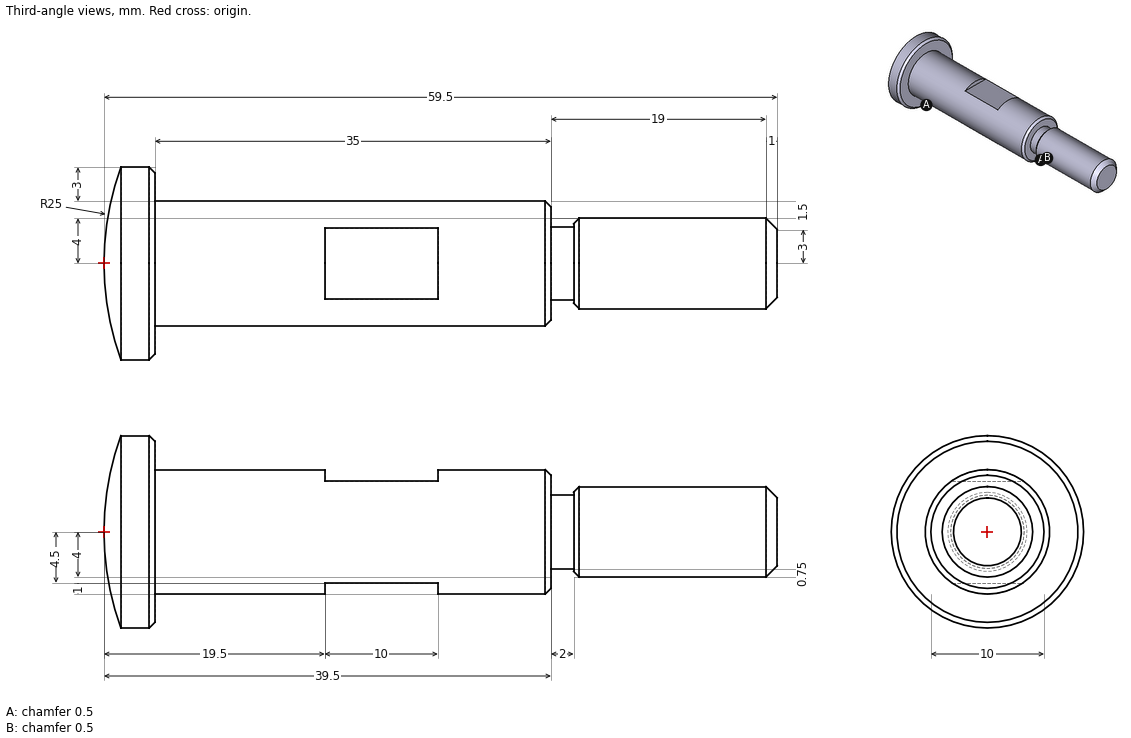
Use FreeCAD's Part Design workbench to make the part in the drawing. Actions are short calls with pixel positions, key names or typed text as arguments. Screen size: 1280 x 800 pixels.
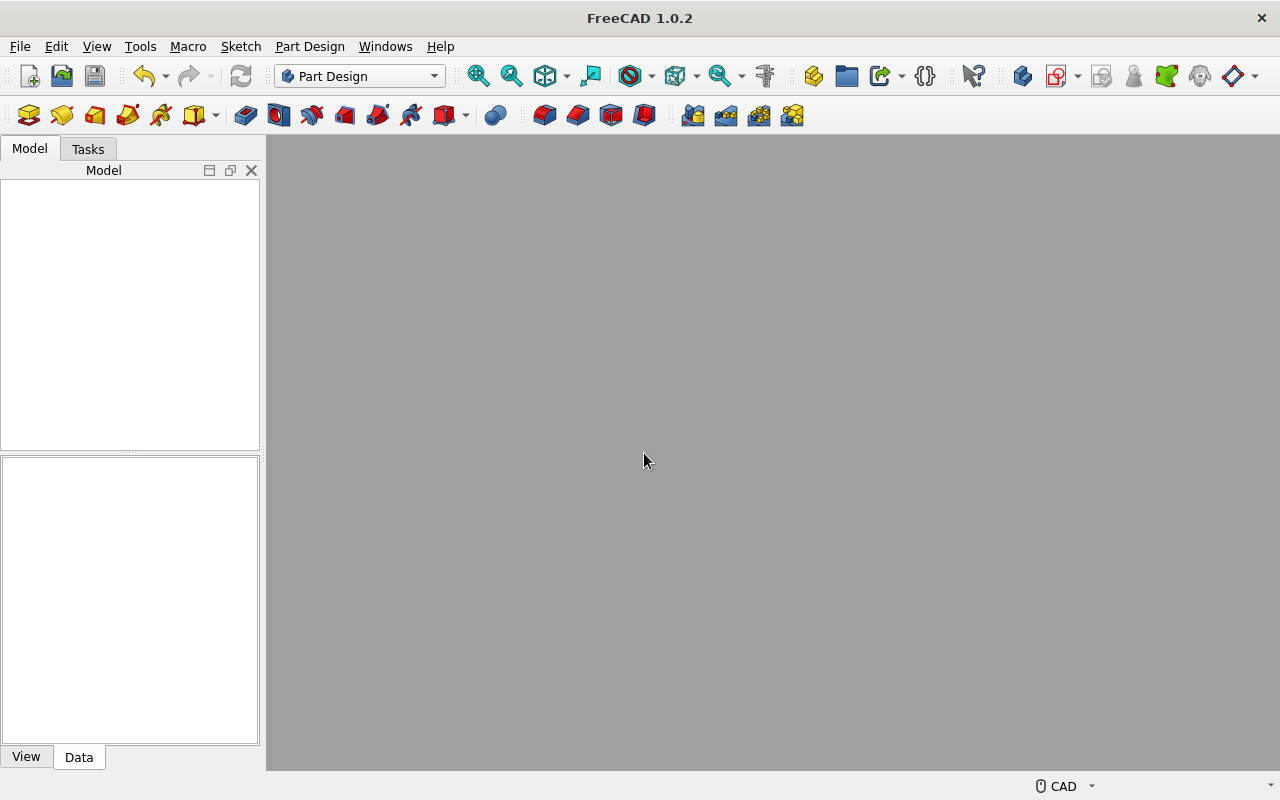
click(29, 76)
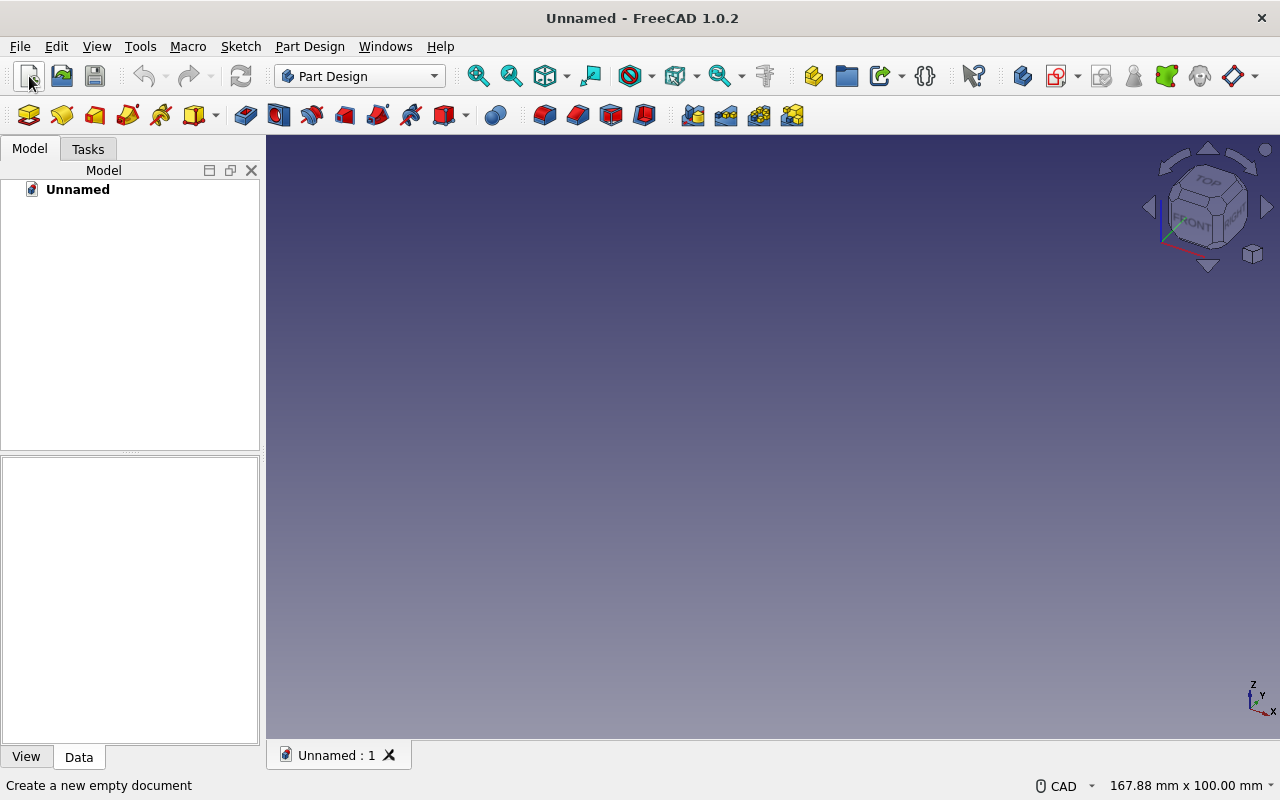
click(1056, 76)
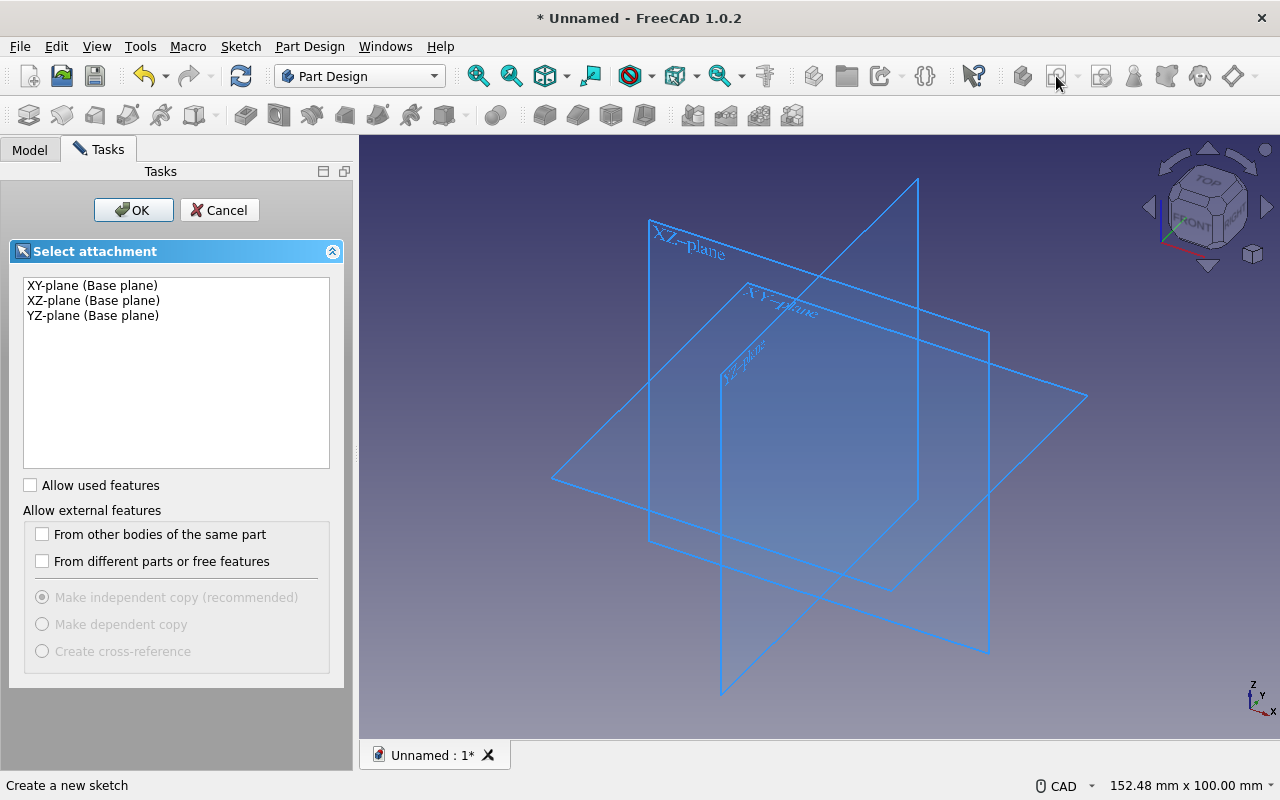
click(84, 286)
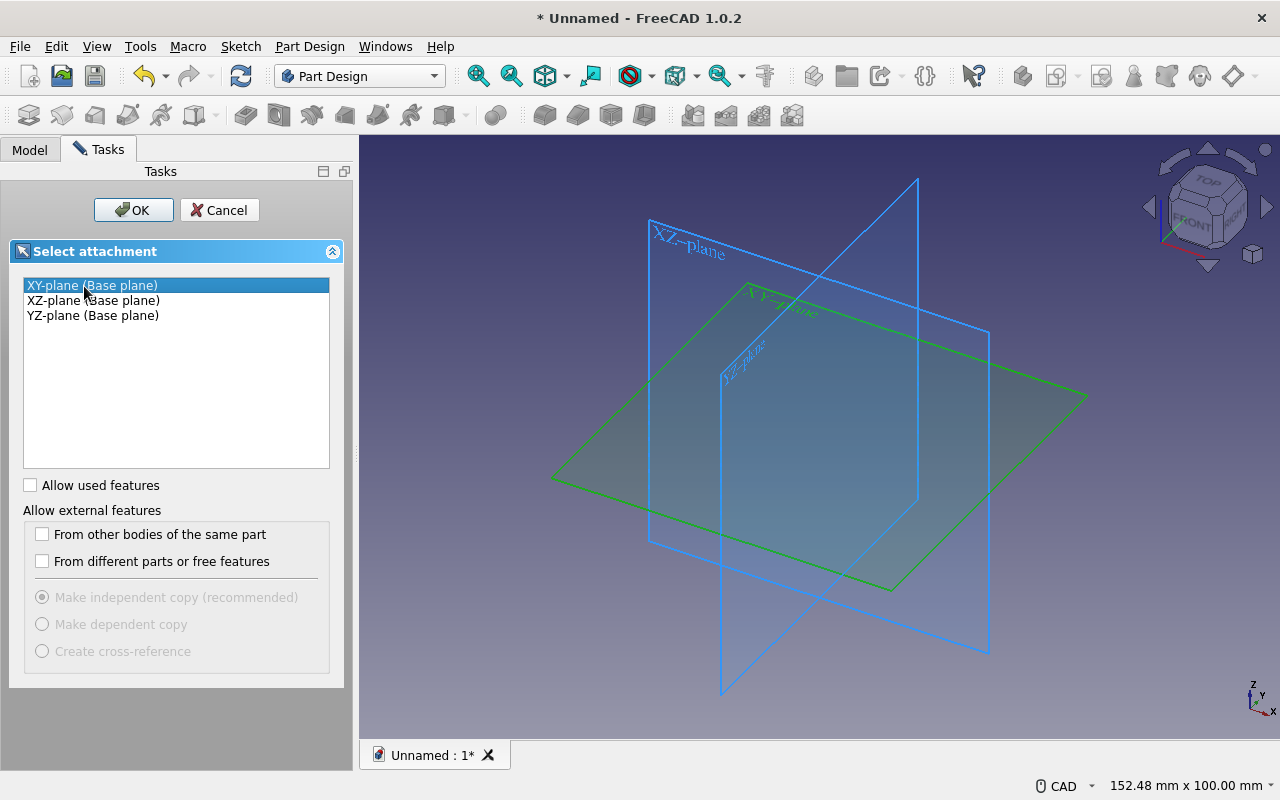
click(134, 210)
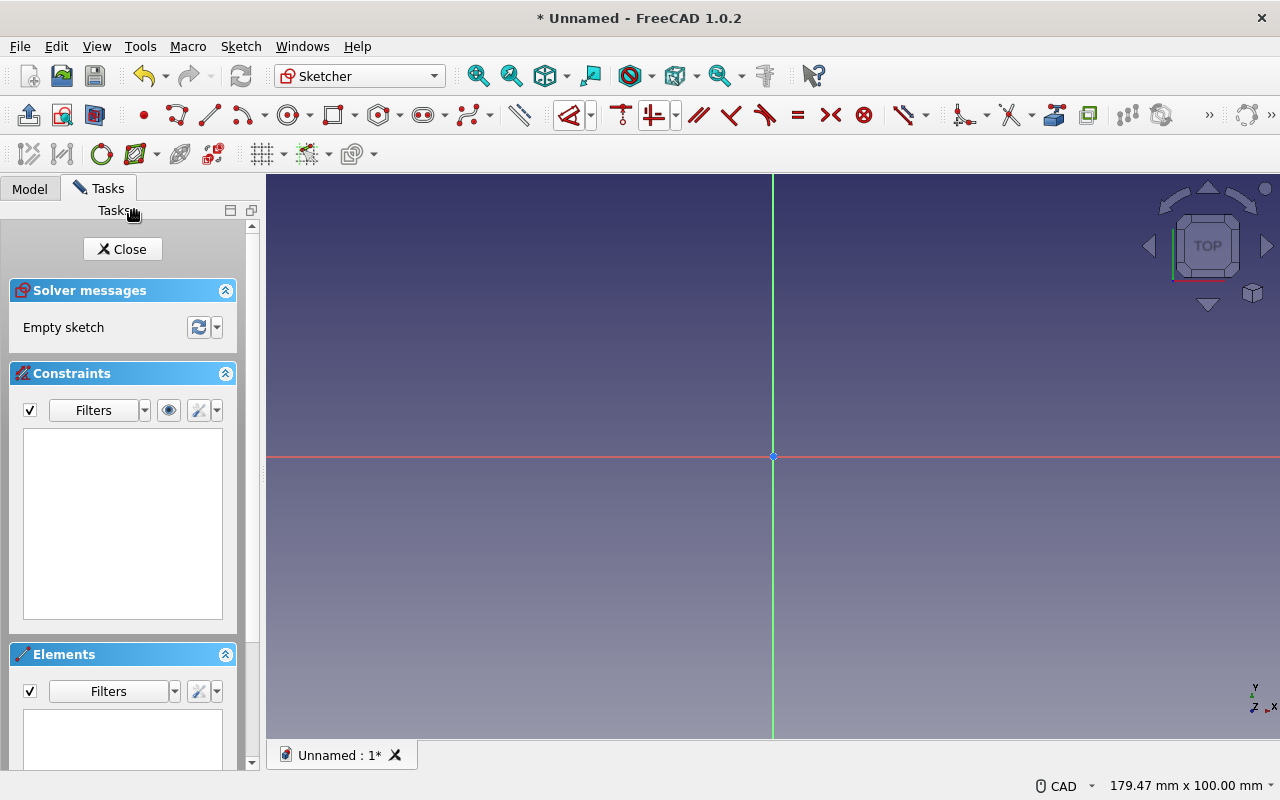
scroll(704, 456, down, 5)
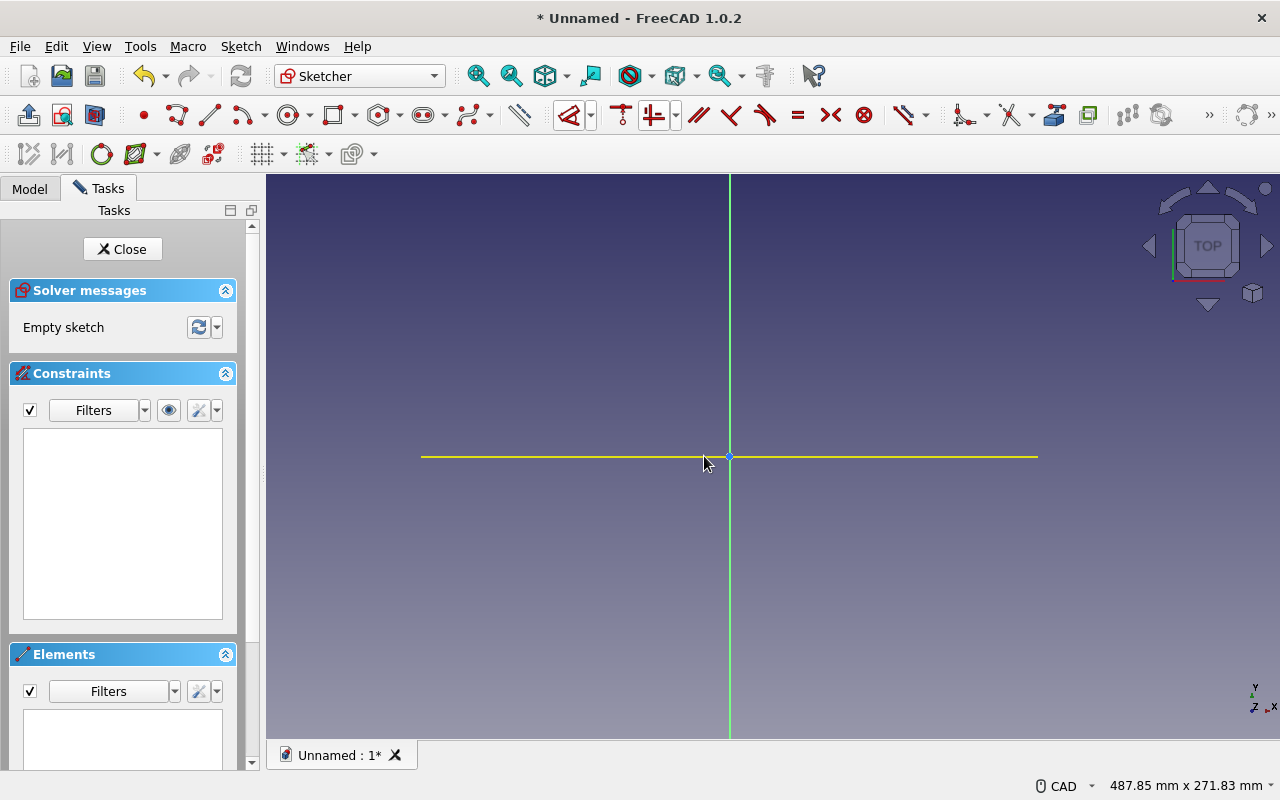
scroll(813, 445, up, 8)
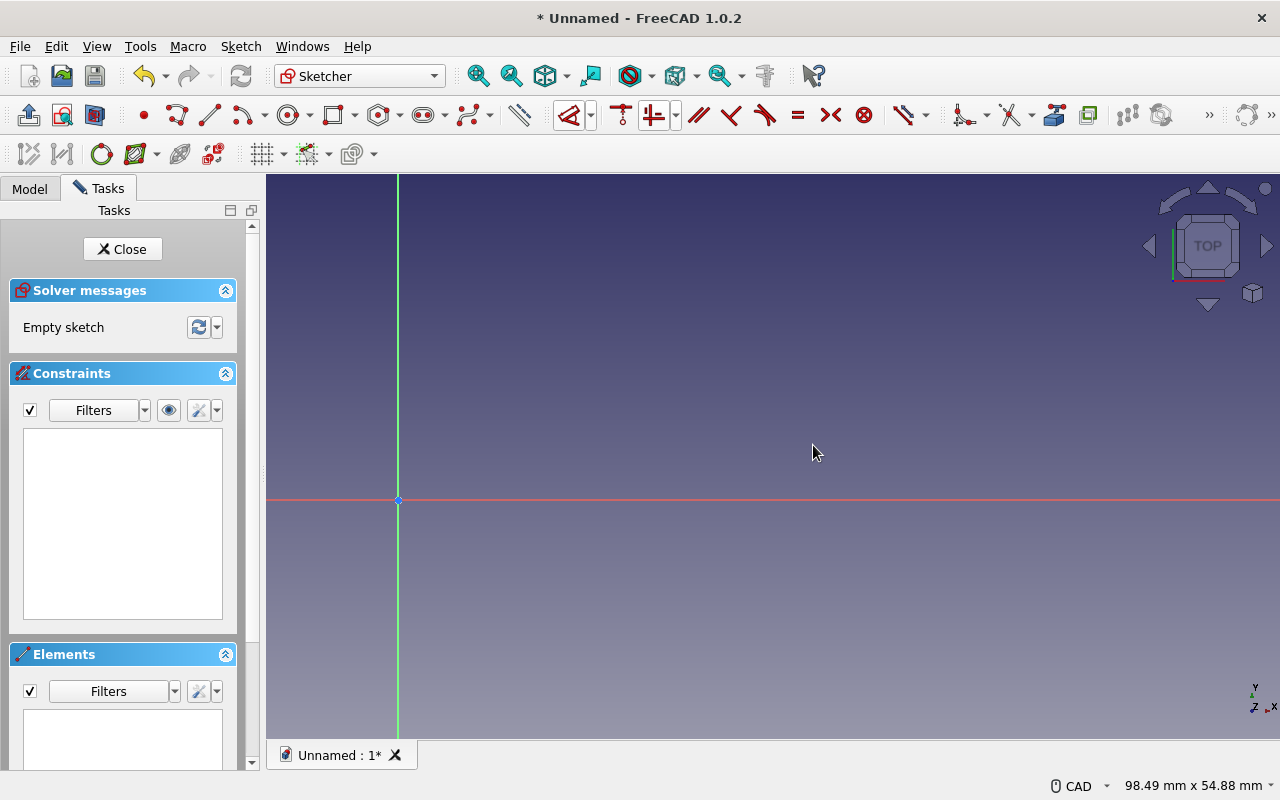
key(g)
key(m)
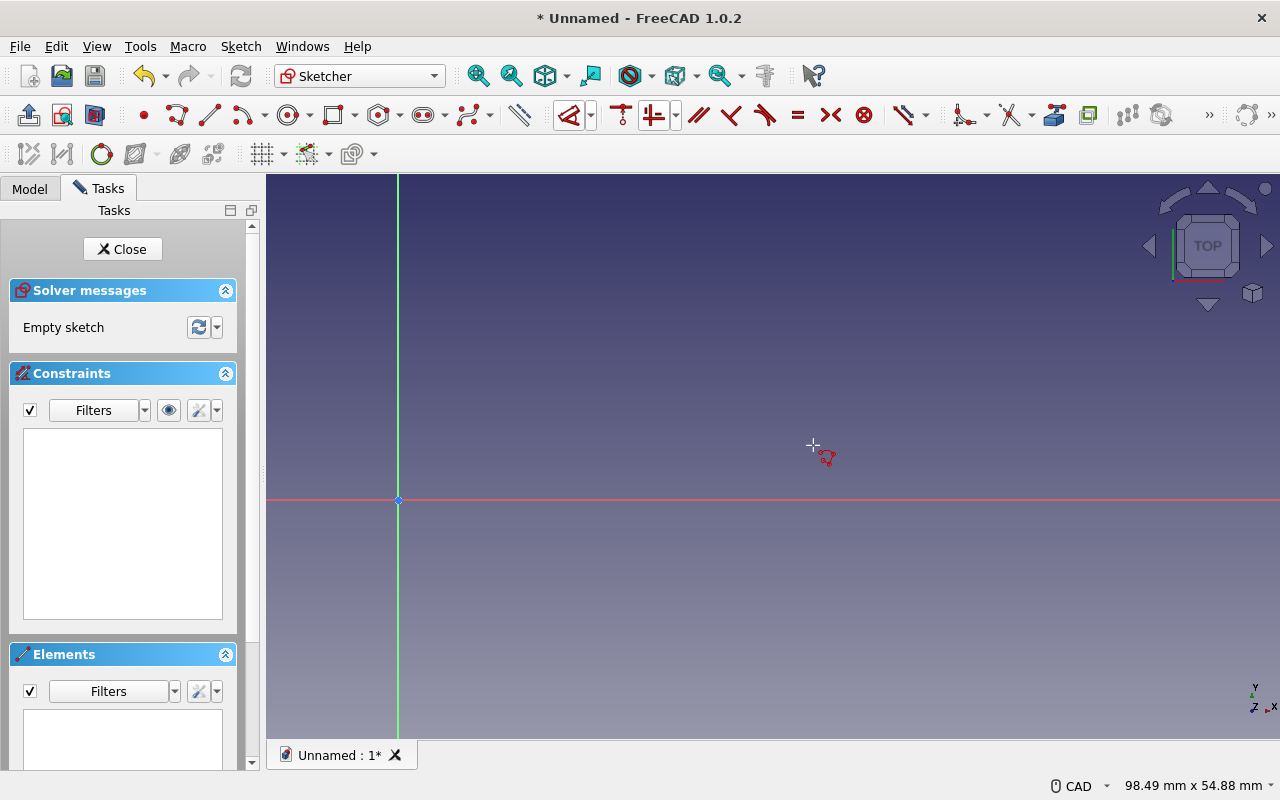
click(398, 500)
click(1011, 491)
click(1011, 469)
click(1000, 459)
click(805, 459)
click(805, 443)
click(444, 443)
click(444, 413)
click(413, 413)
right_click(413, 413)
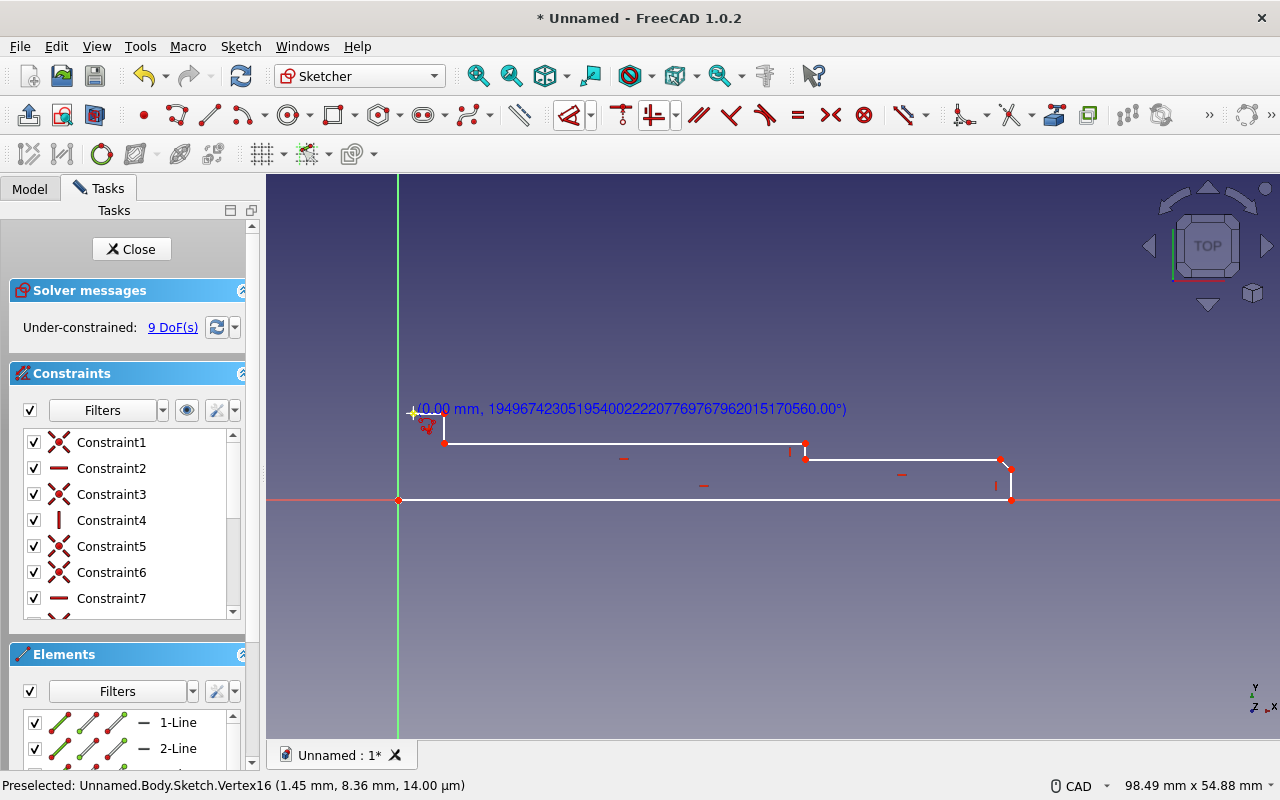
key(g)
key(3)
key(a)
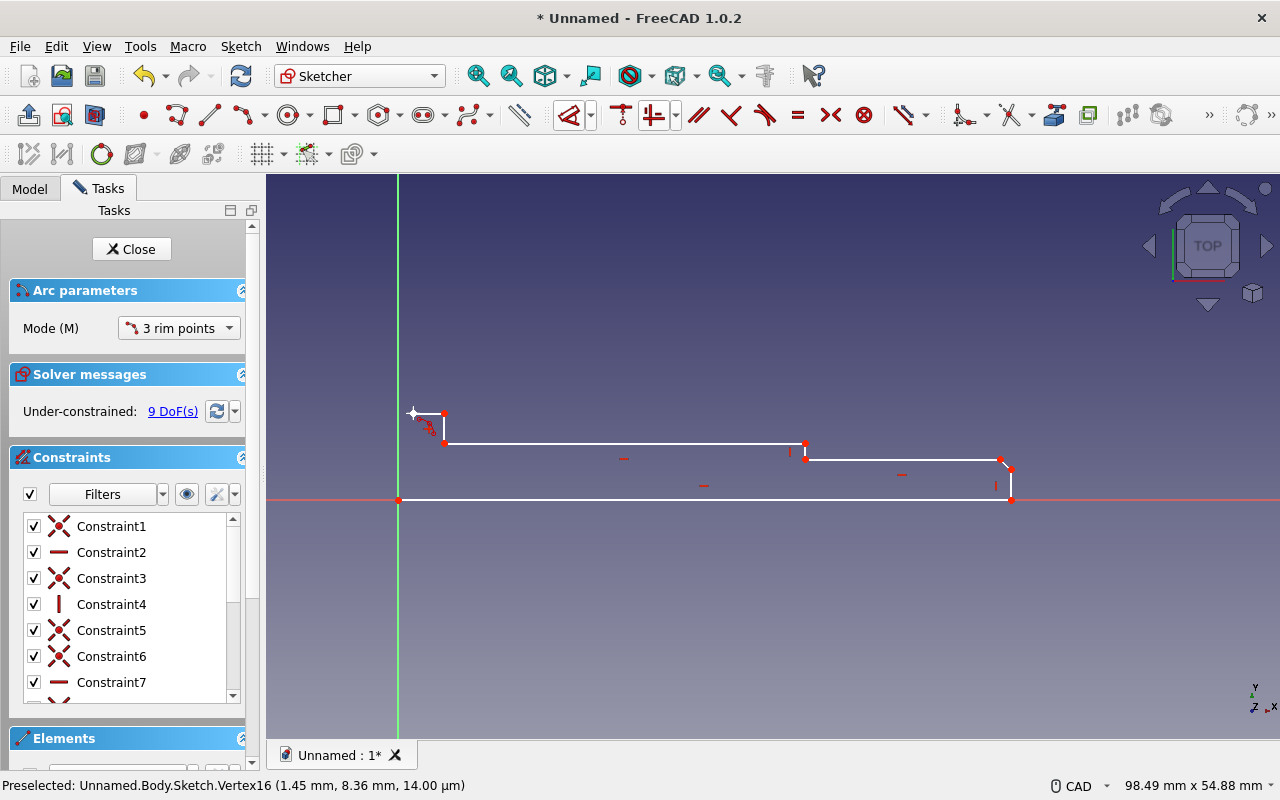
click(413, 414)
click(398, 500)